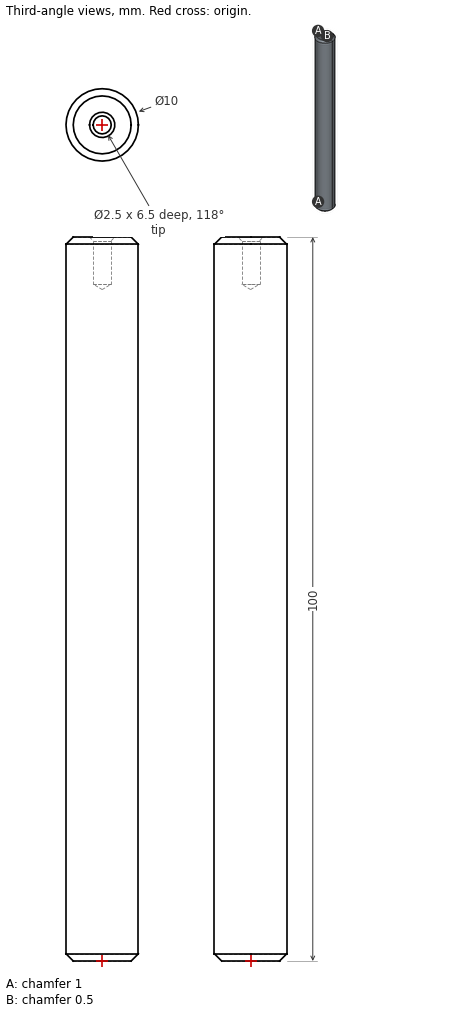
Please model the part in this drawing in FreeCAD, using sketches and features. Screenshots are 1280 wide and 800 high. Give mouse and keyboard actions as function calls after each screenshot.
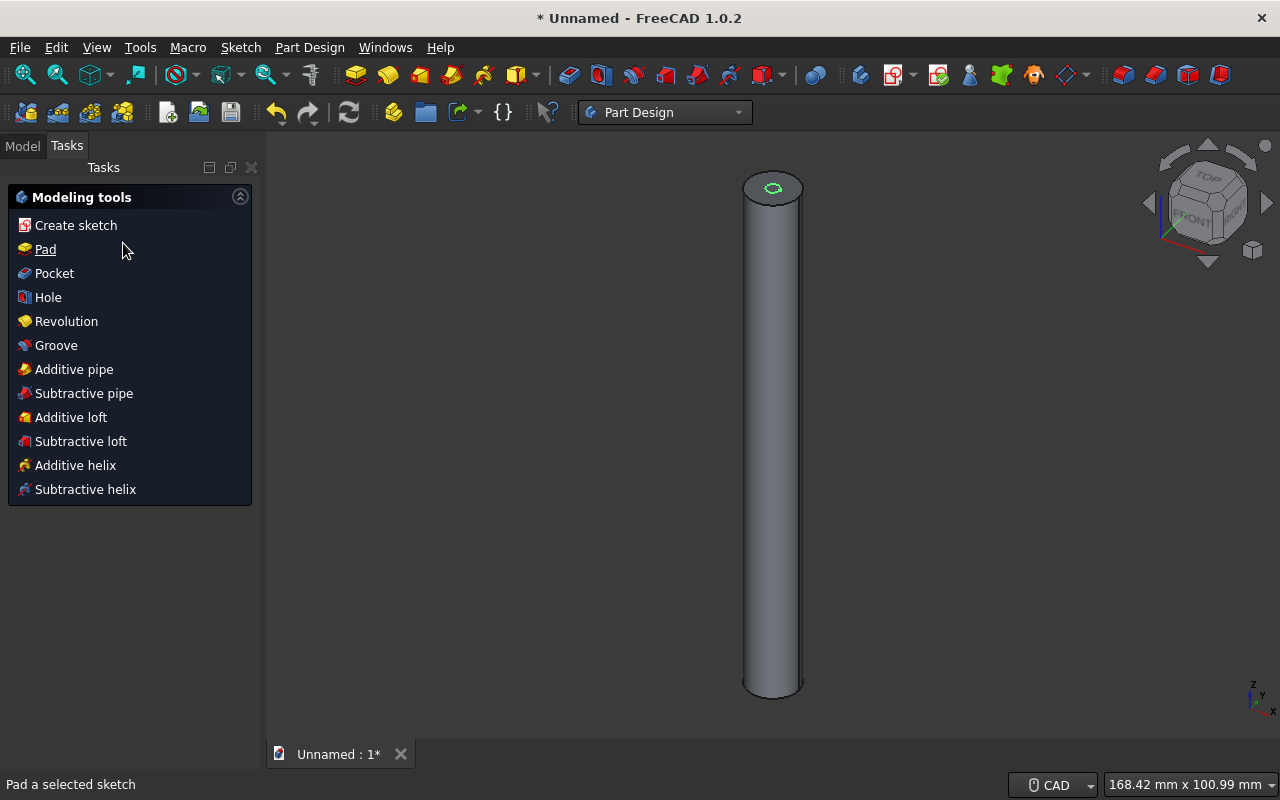
click(602, 76)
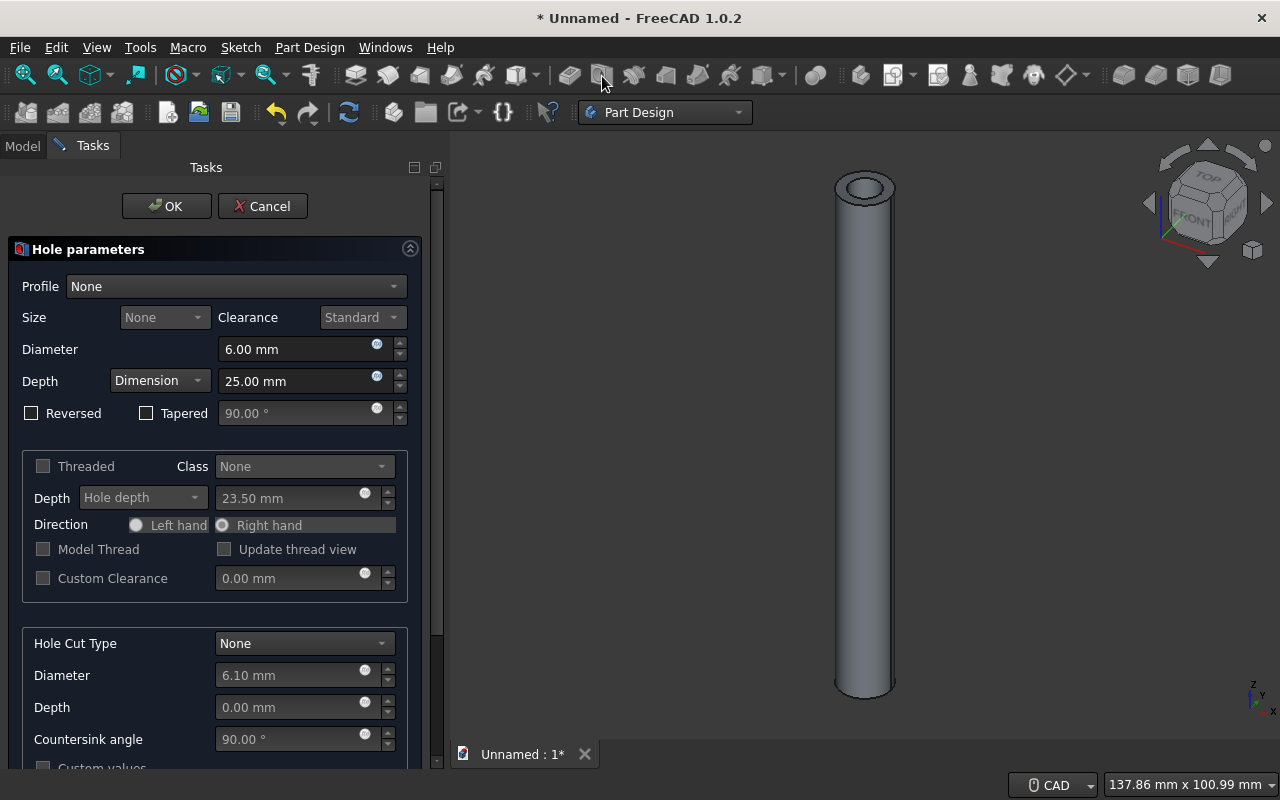
triple_click(305, 349)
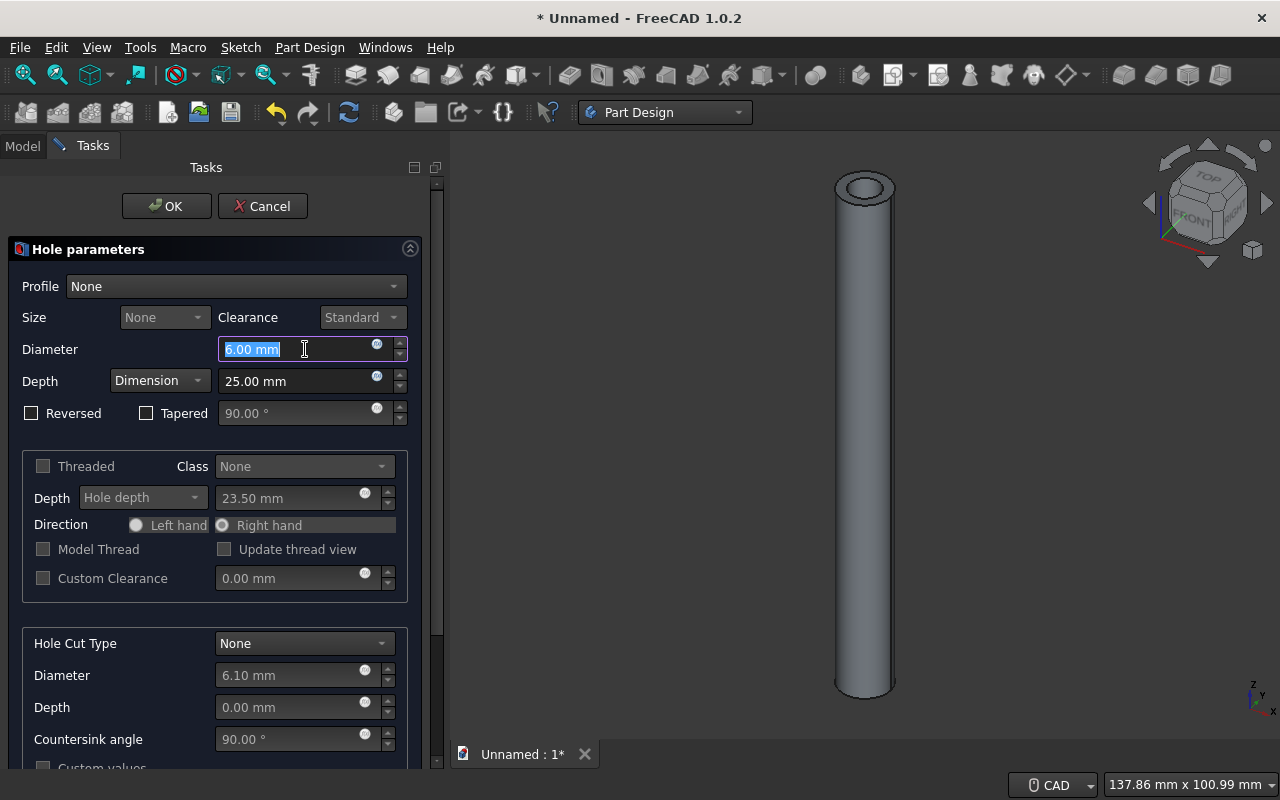
text(2.5)
key(Tab)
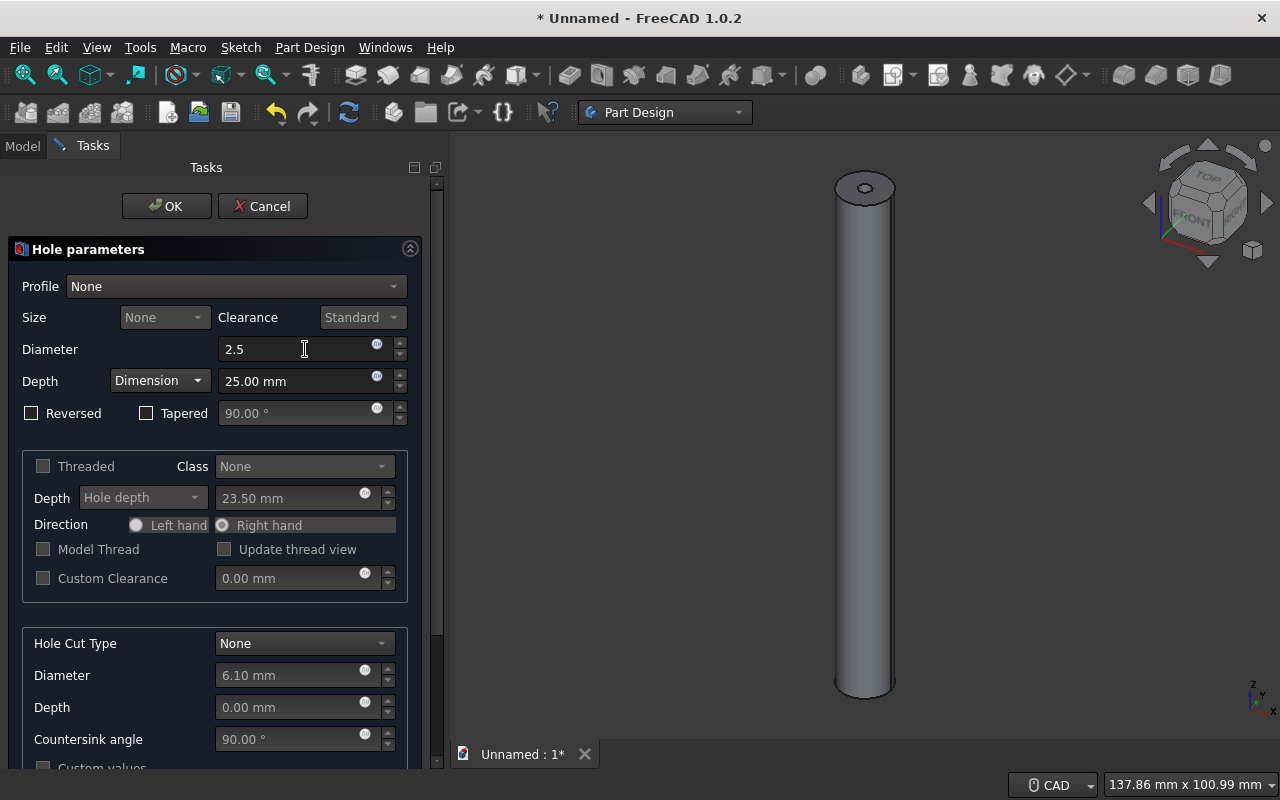
triple_click(305, 381)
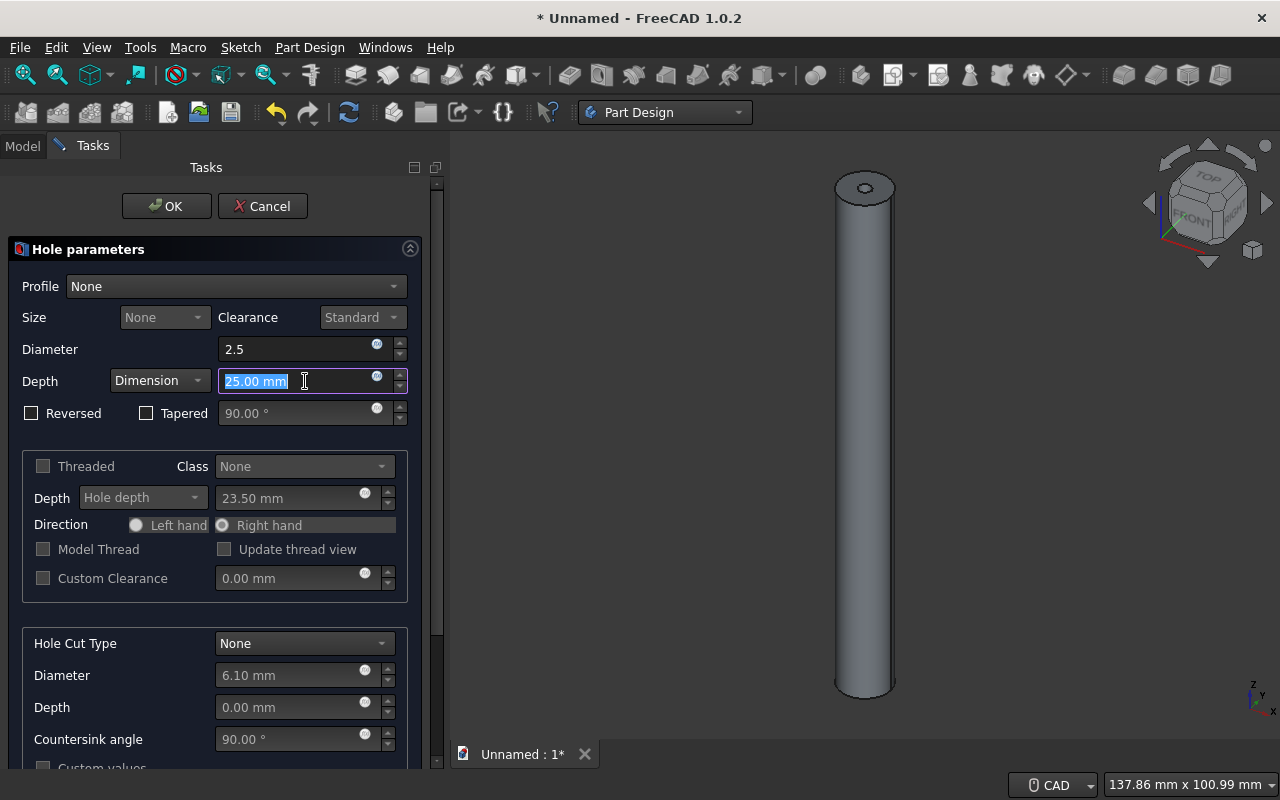
text(6.5)
key(Tab)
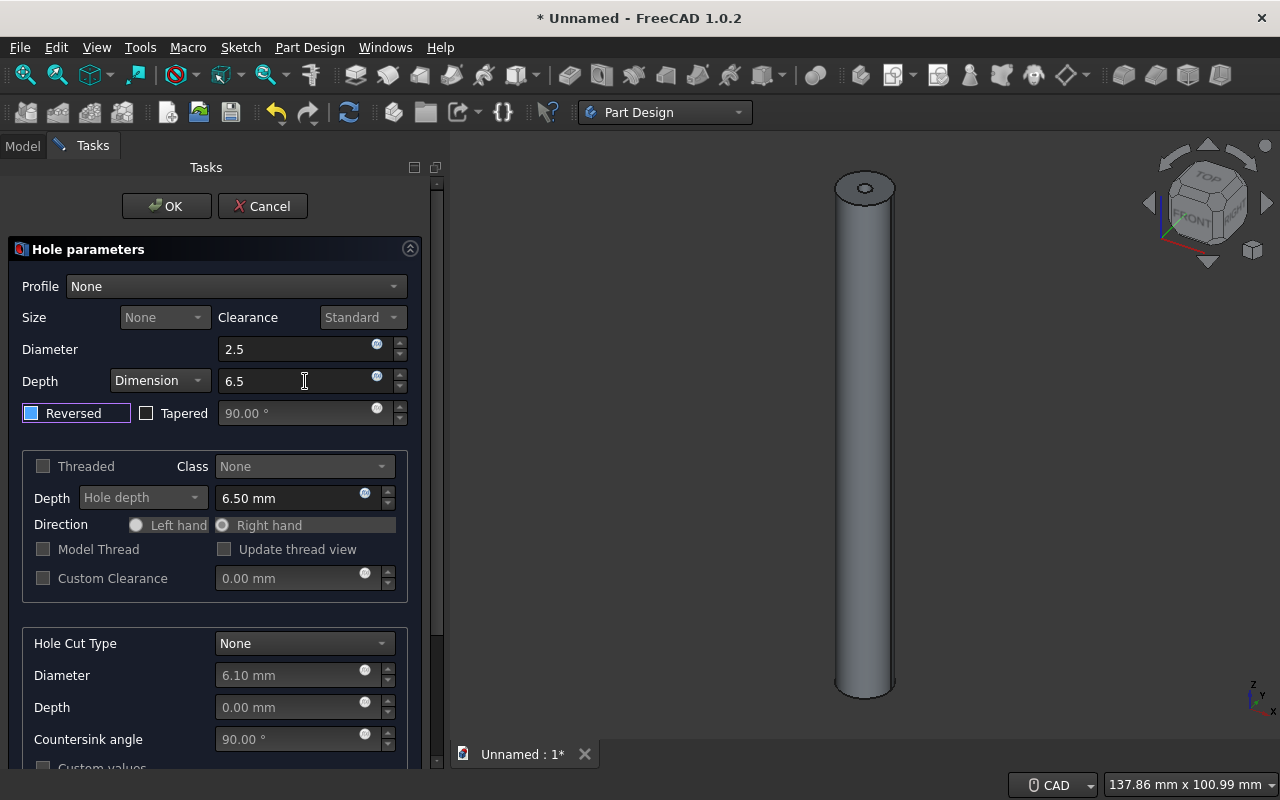
click(167, 206)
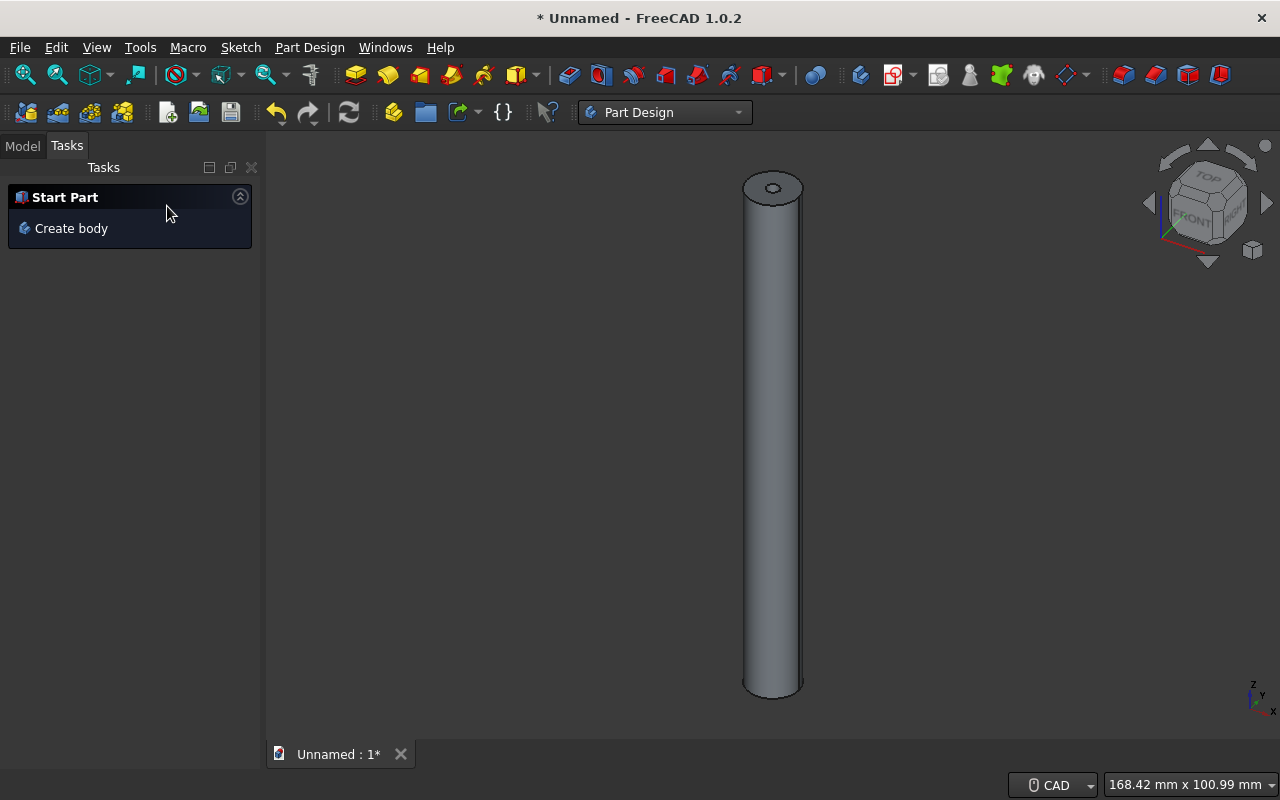
click(743, 189)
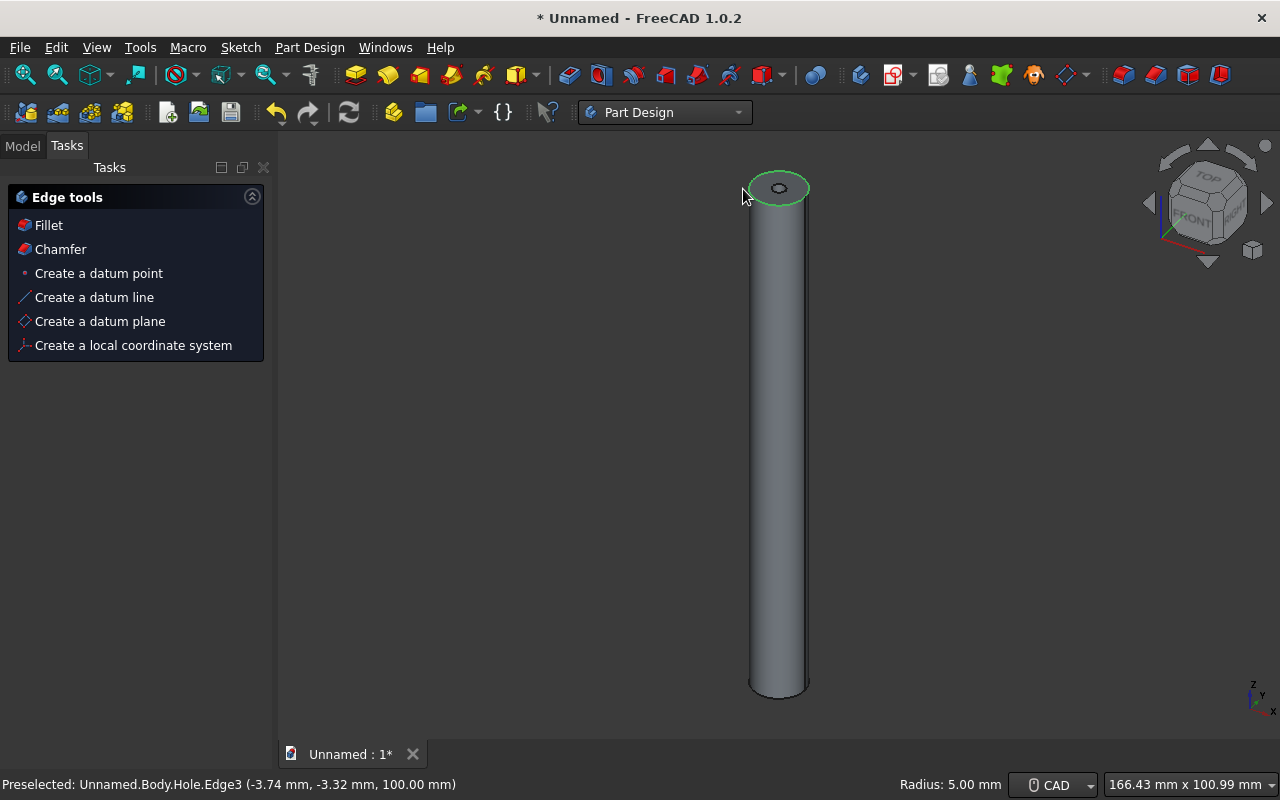
key(0)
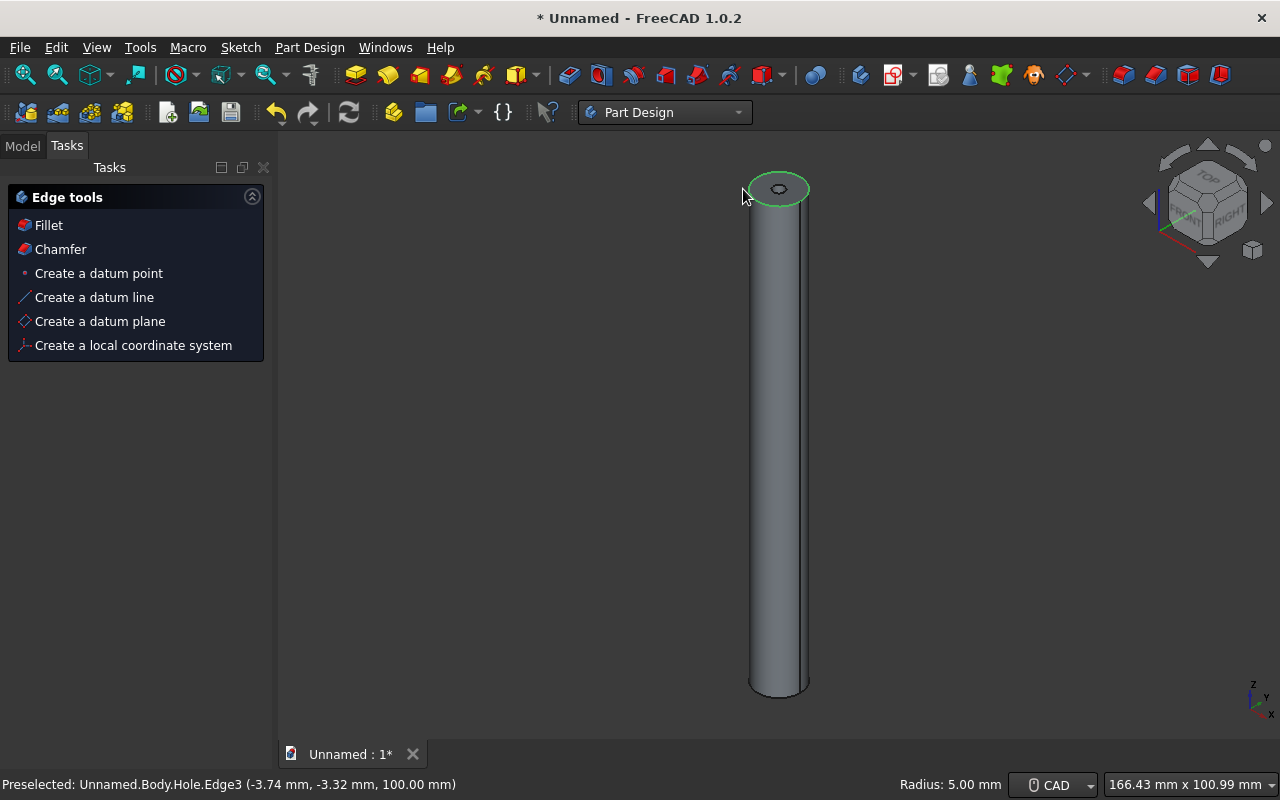
click(752, 688, ctrl)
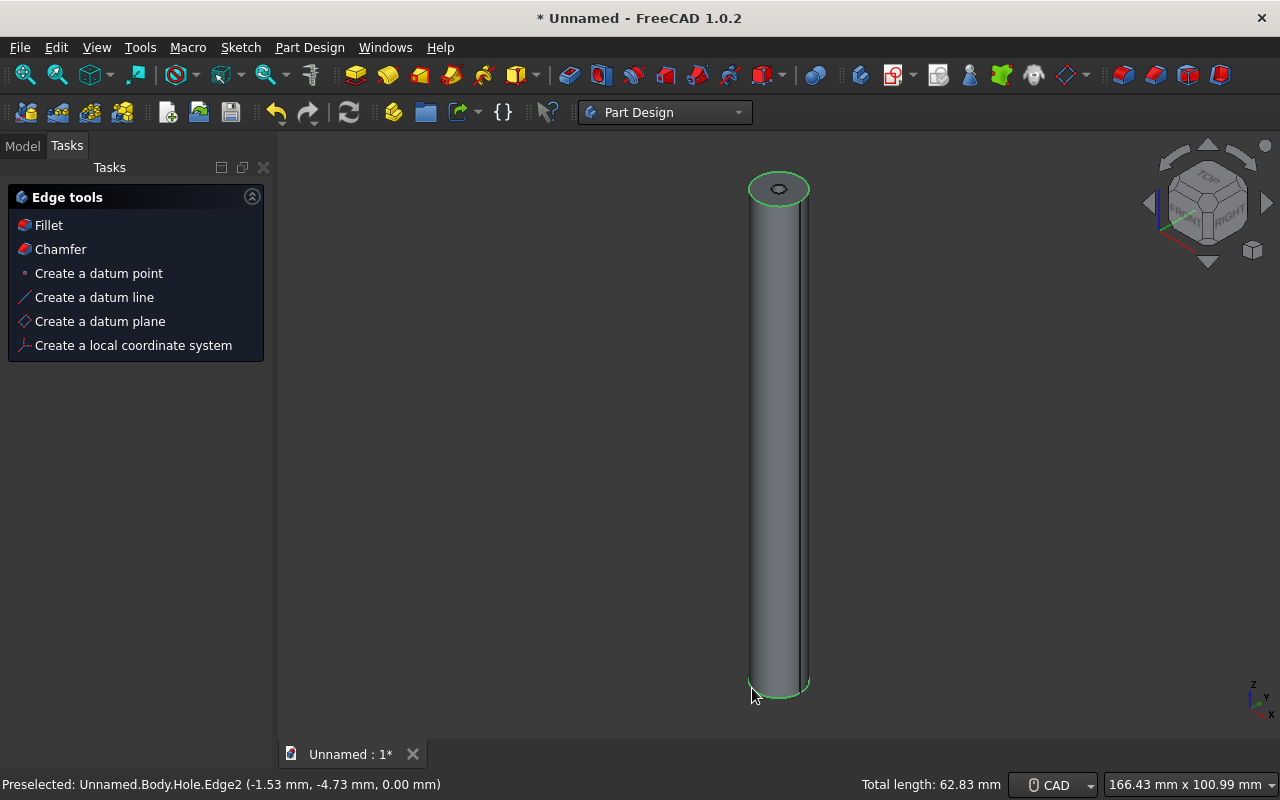
click(1156, 76)